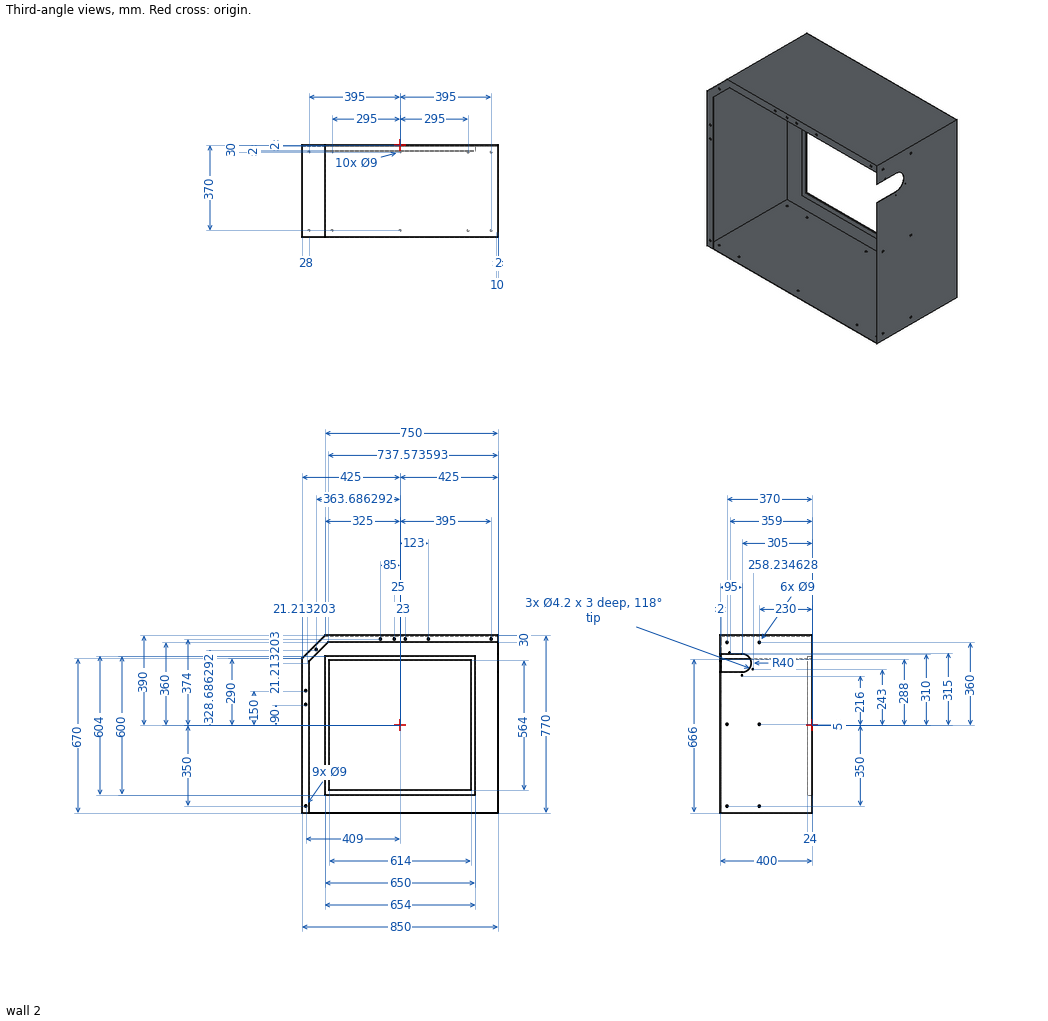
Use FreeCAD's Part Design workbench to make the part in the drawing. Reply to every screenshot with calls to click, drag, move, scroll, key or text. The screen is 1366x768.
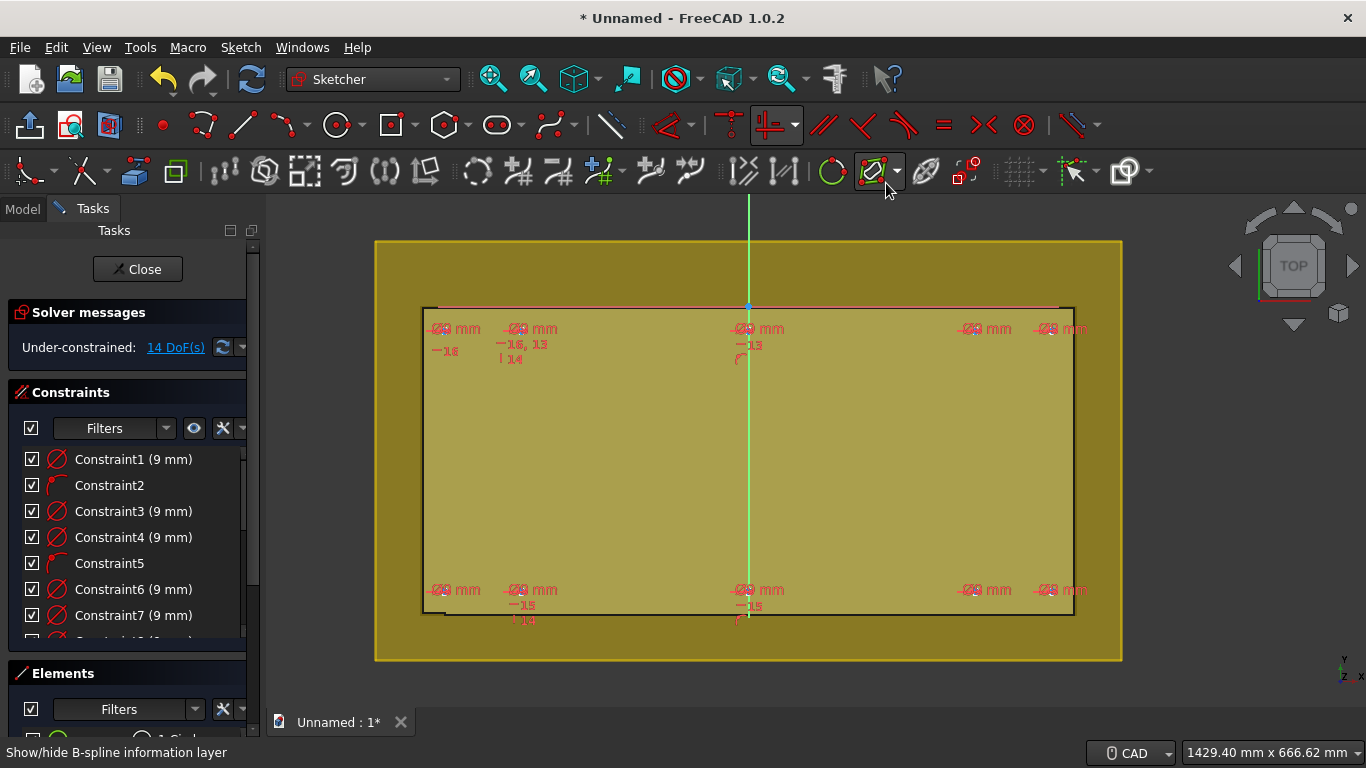
click(445, 331)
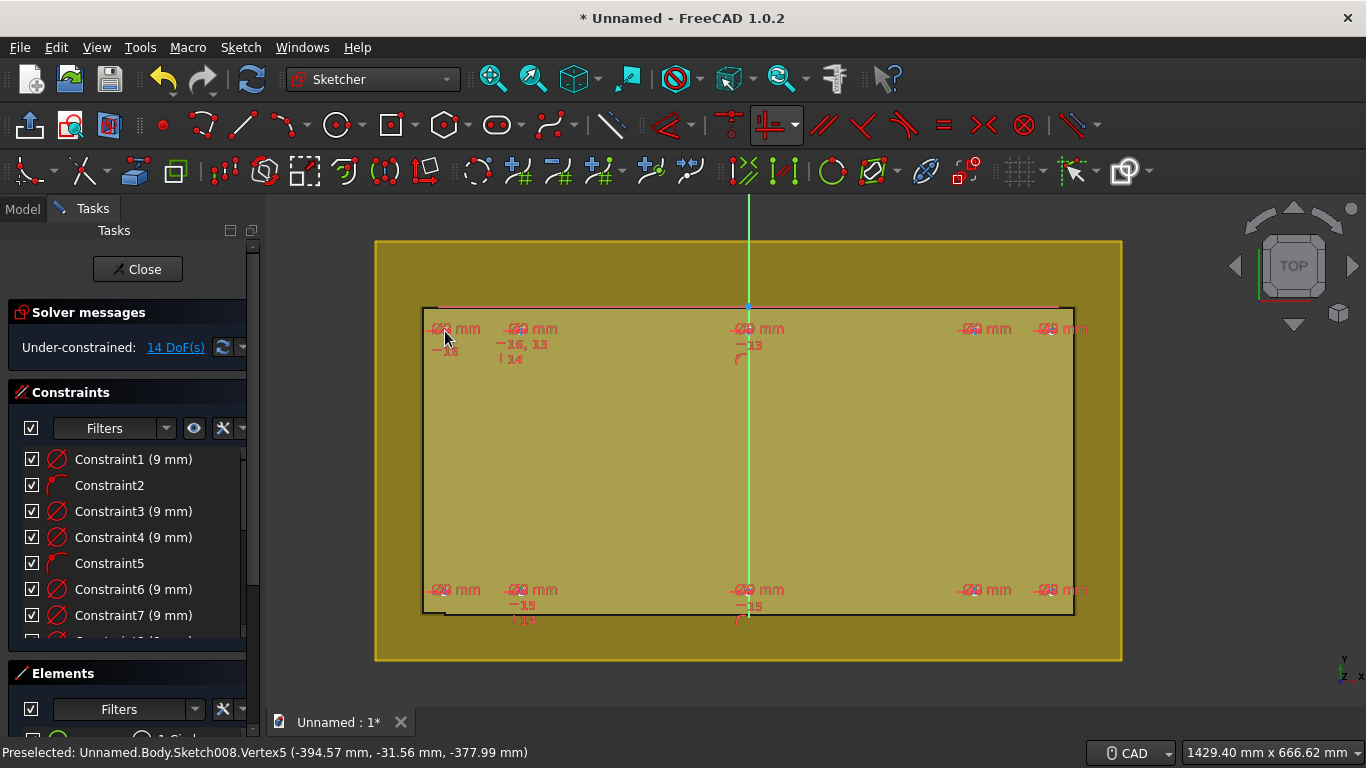
click(445, 592)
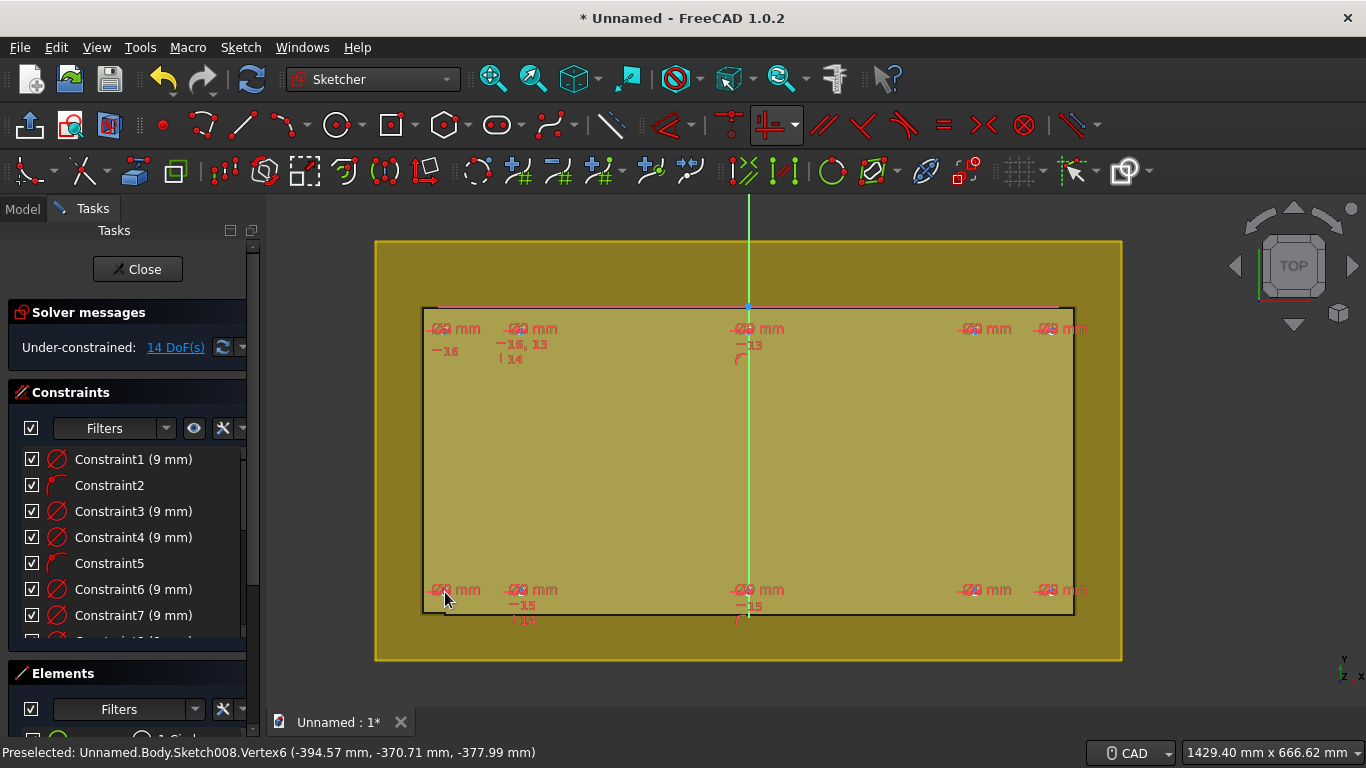
key(v)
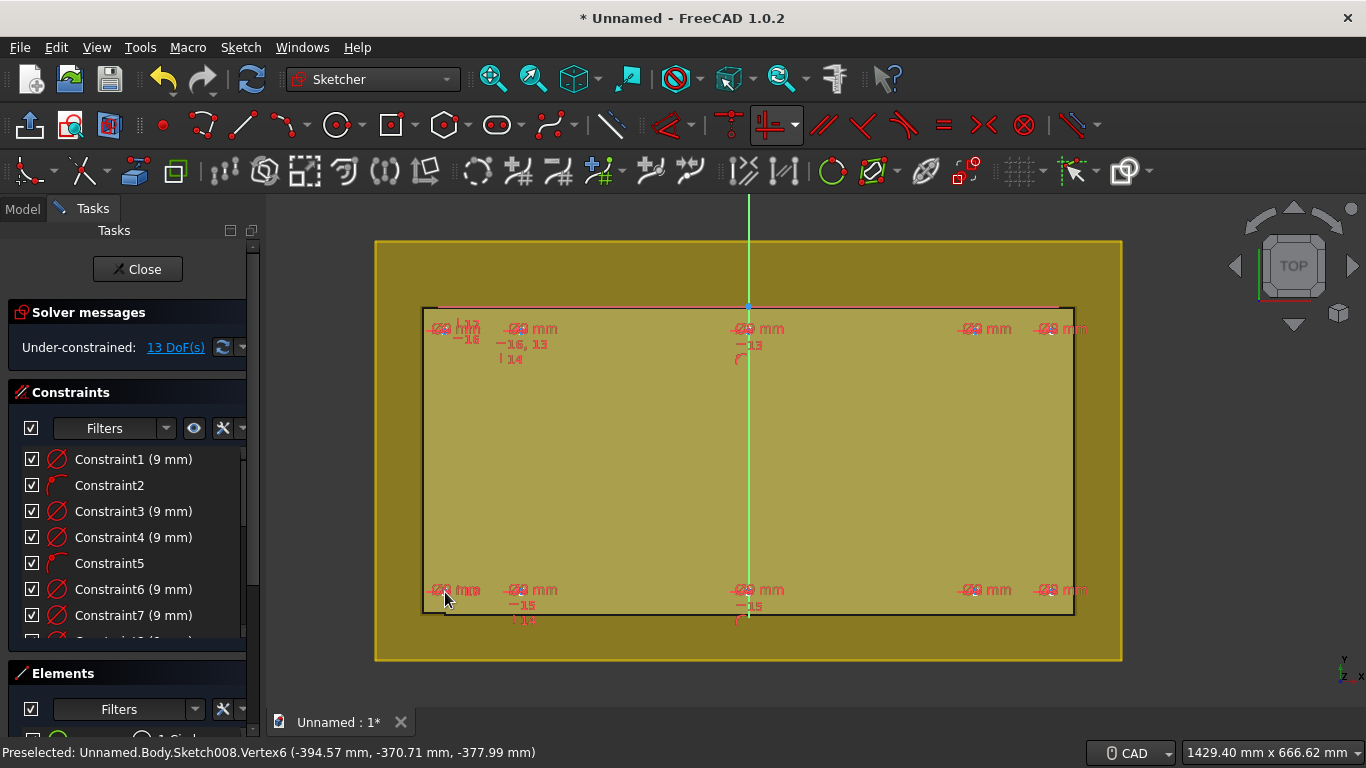
click(522, 592)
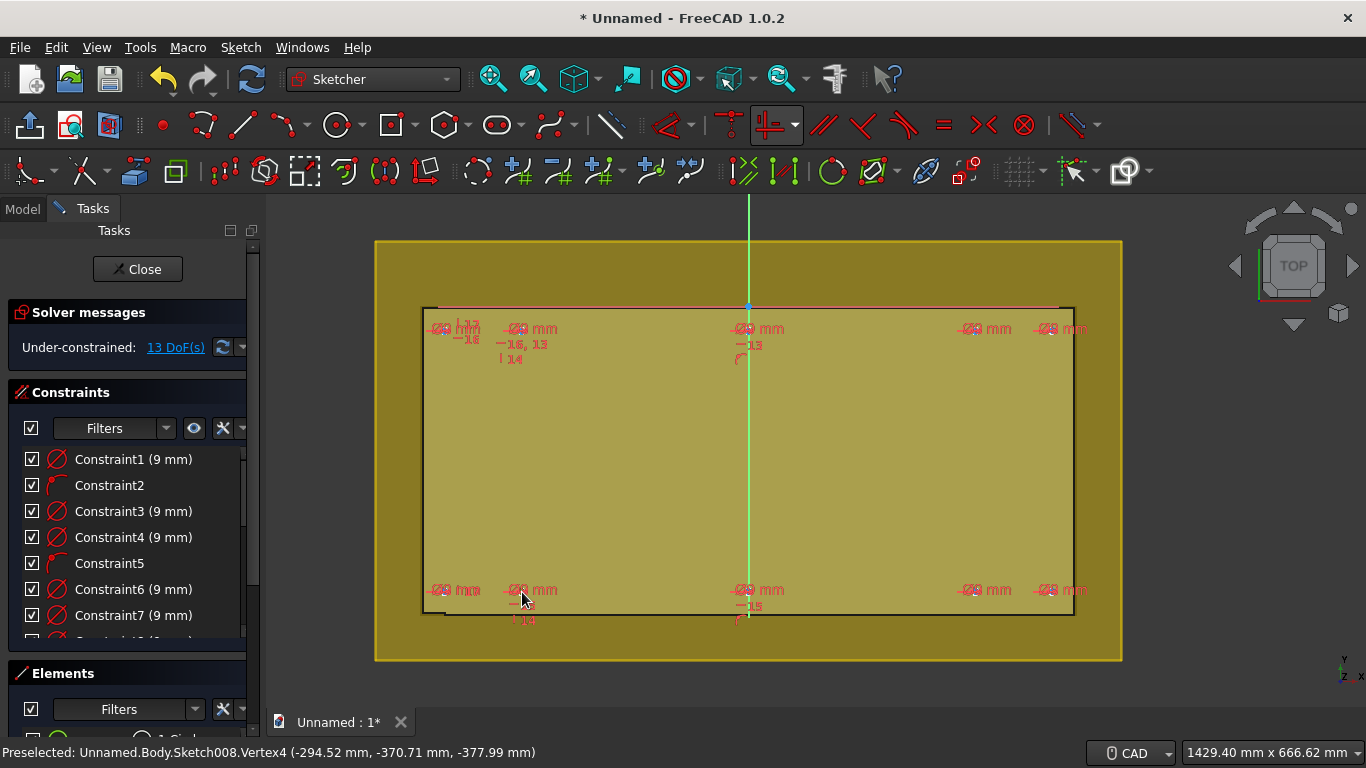
click(445, 592)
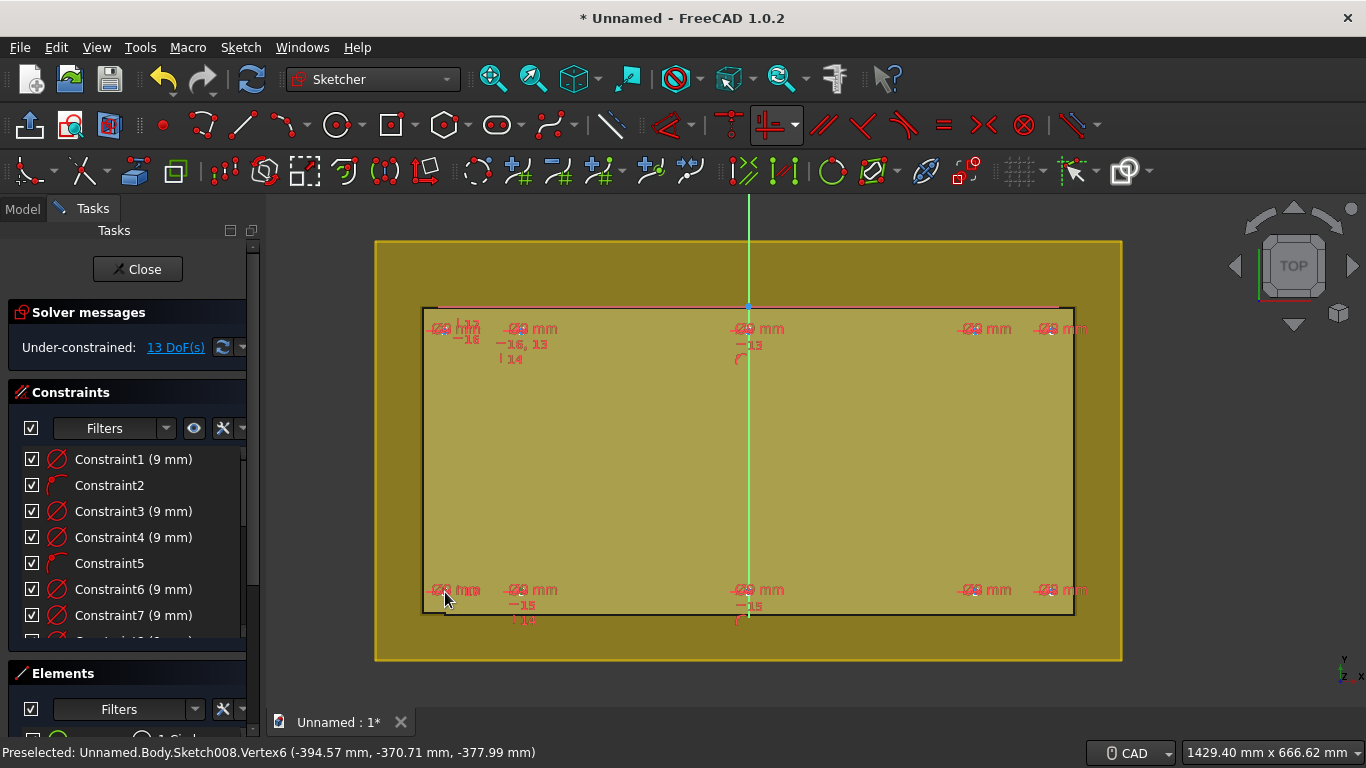
key(h)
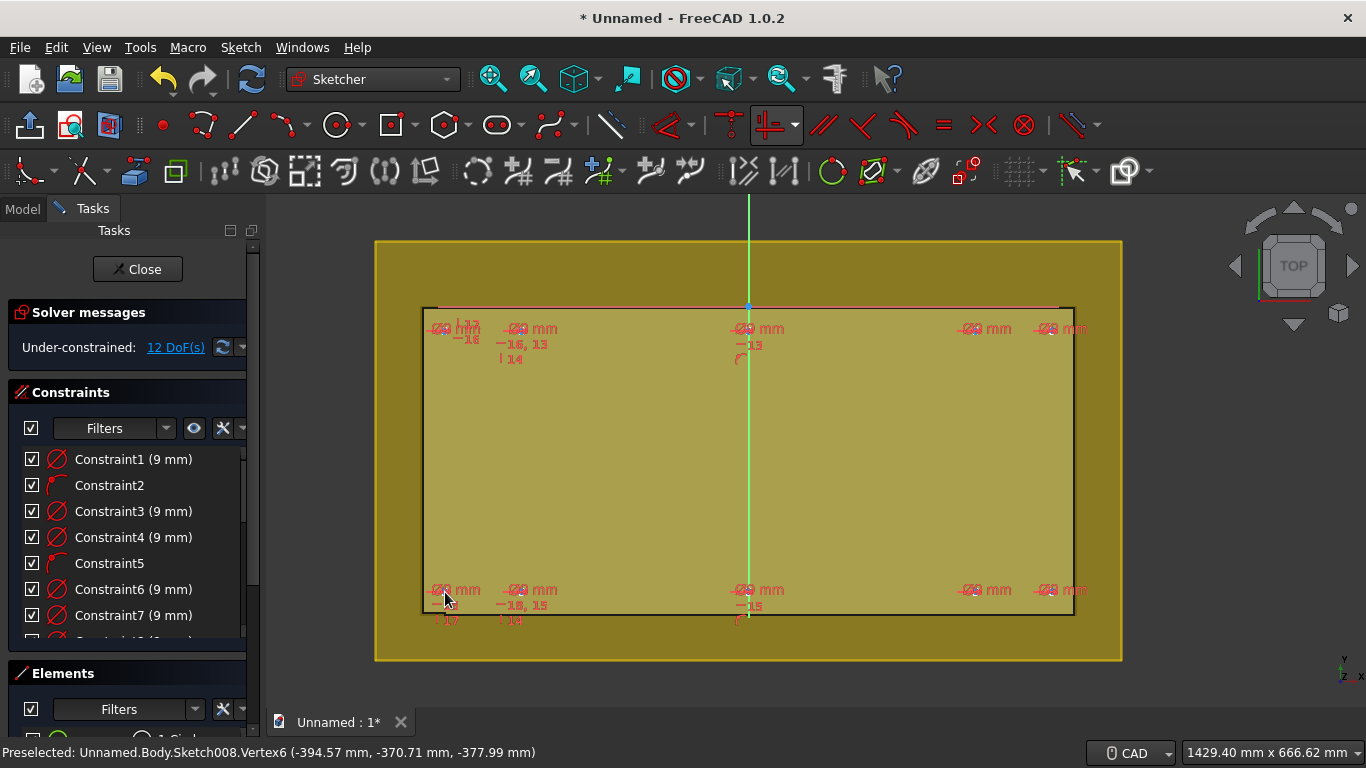
click(749, 331)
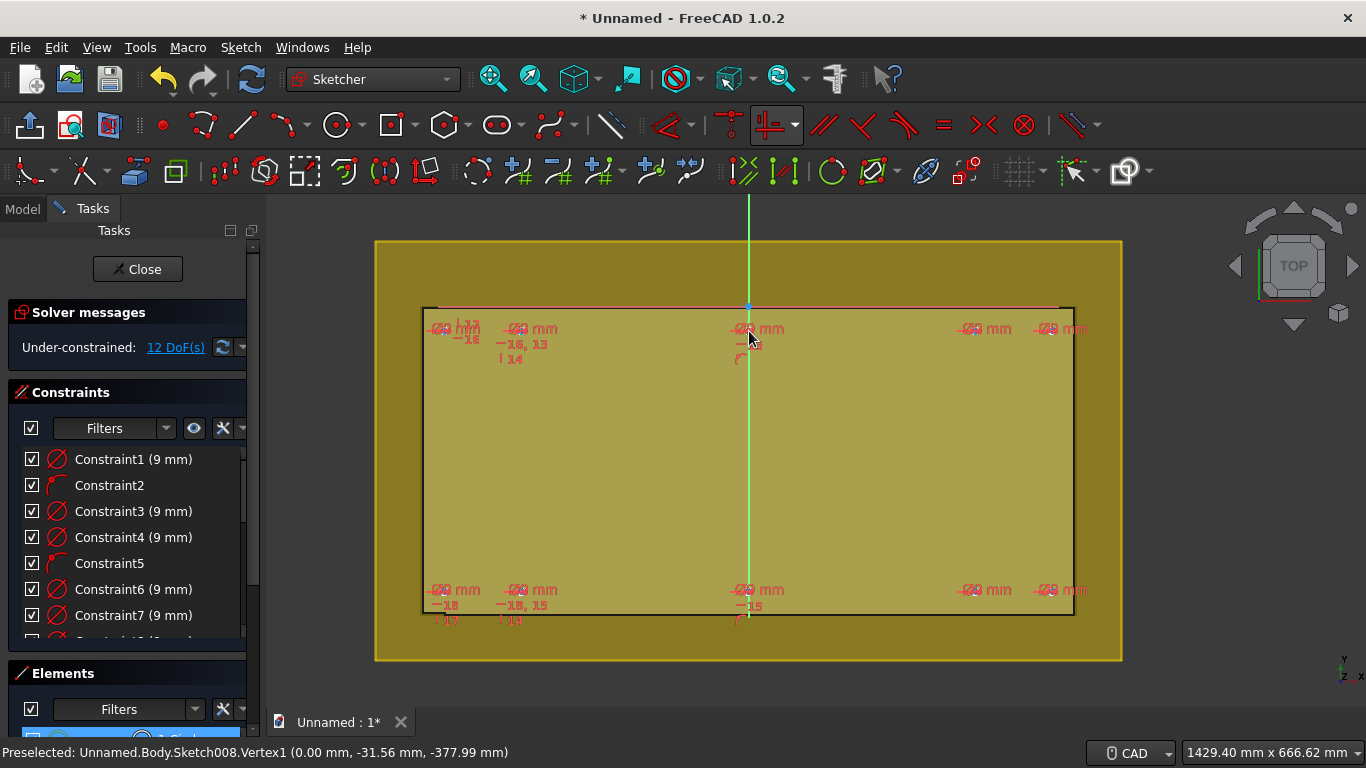
click(976, 331)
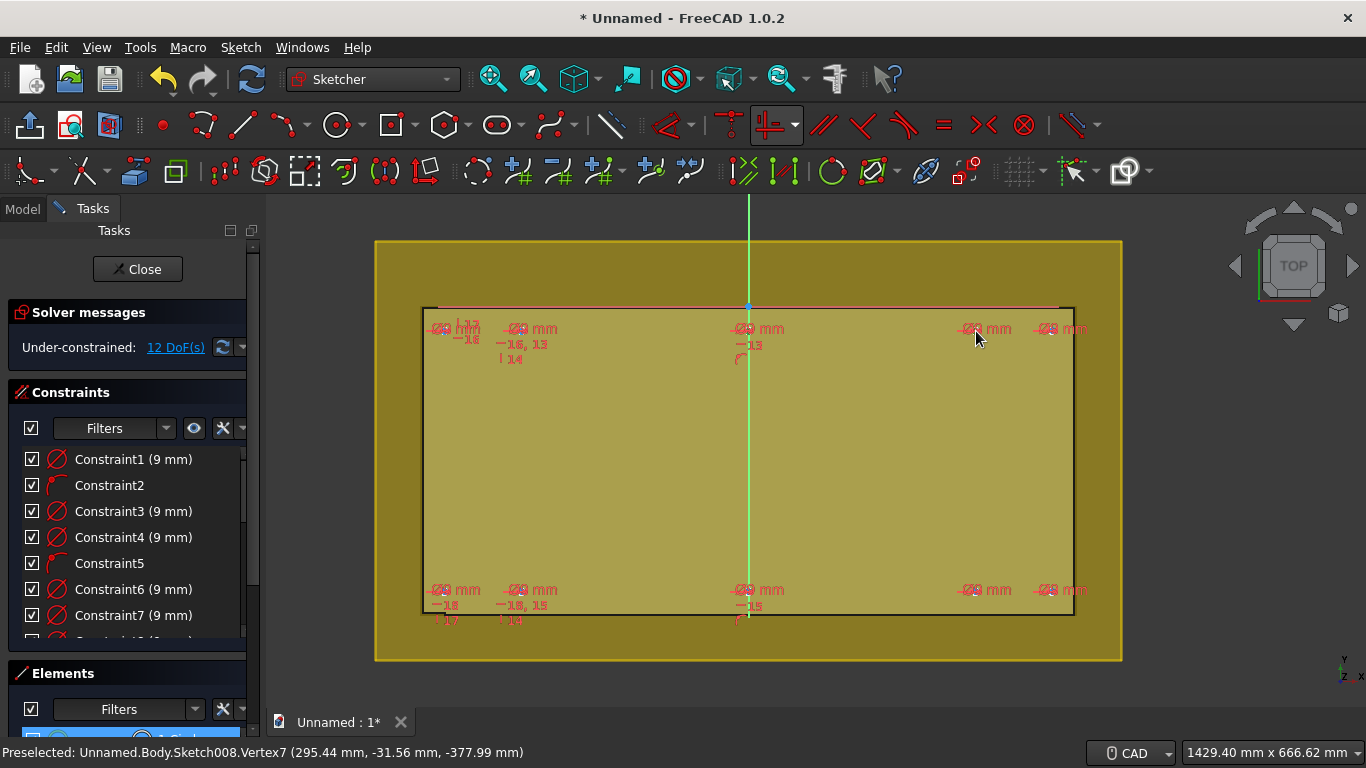
click(798, 126)